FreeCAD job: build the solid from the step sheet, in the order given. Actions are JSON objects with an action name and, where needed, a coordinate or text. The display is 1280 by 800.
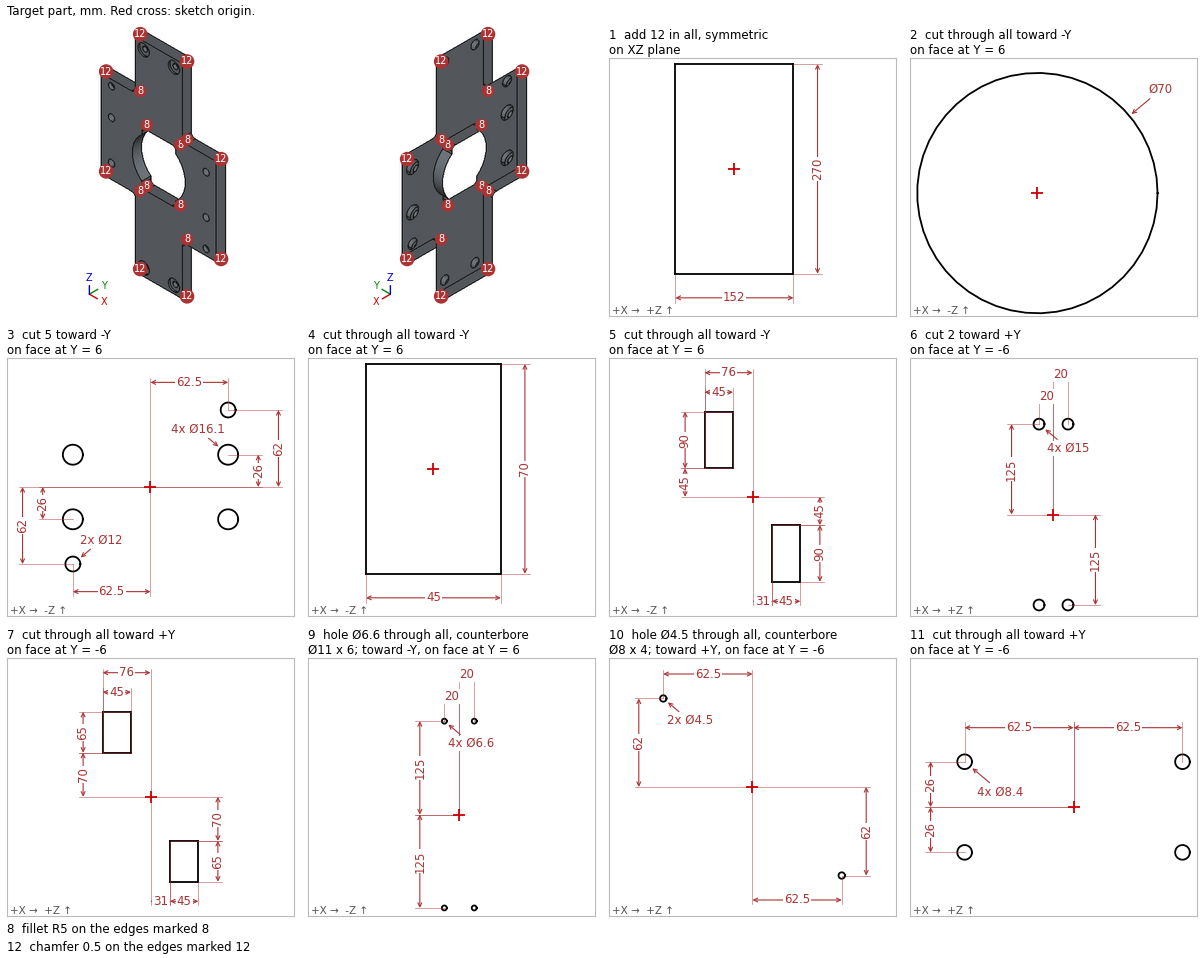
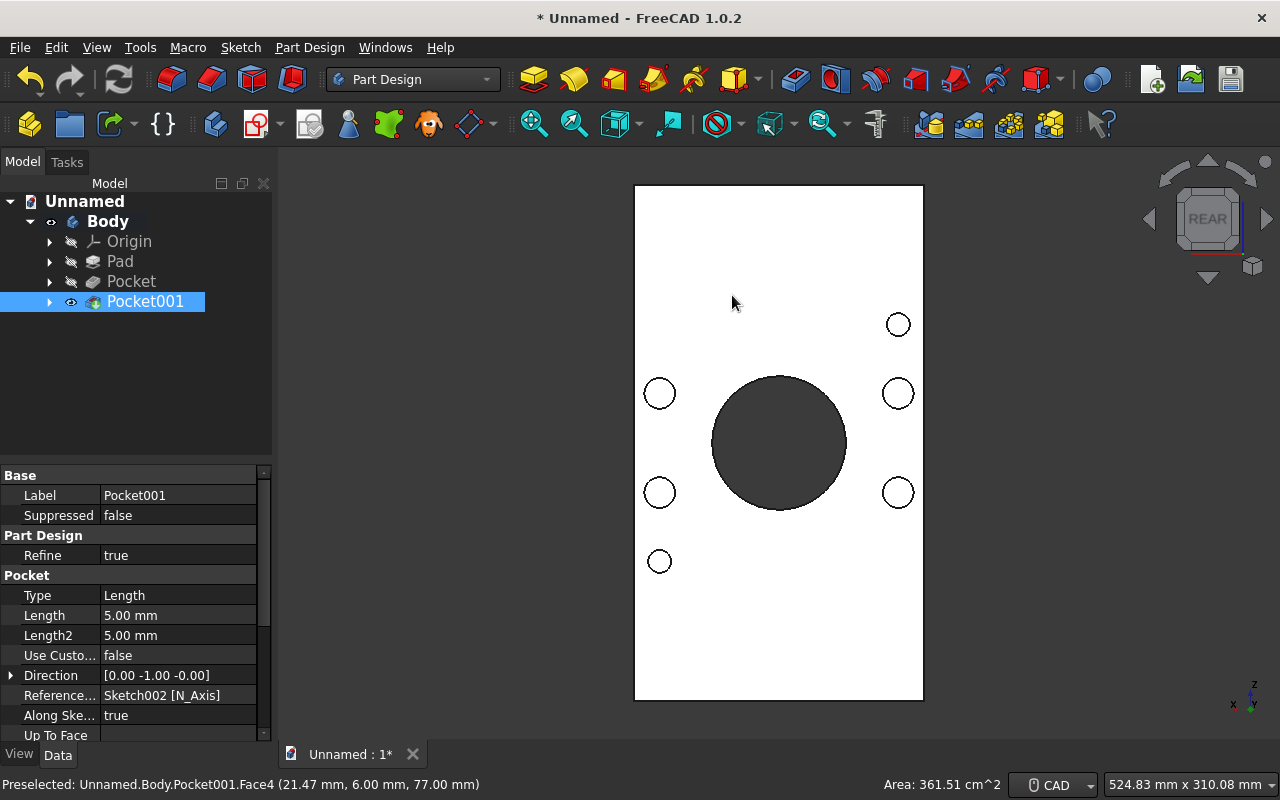
{"action": "left_click", "coordinate": [256, 124]}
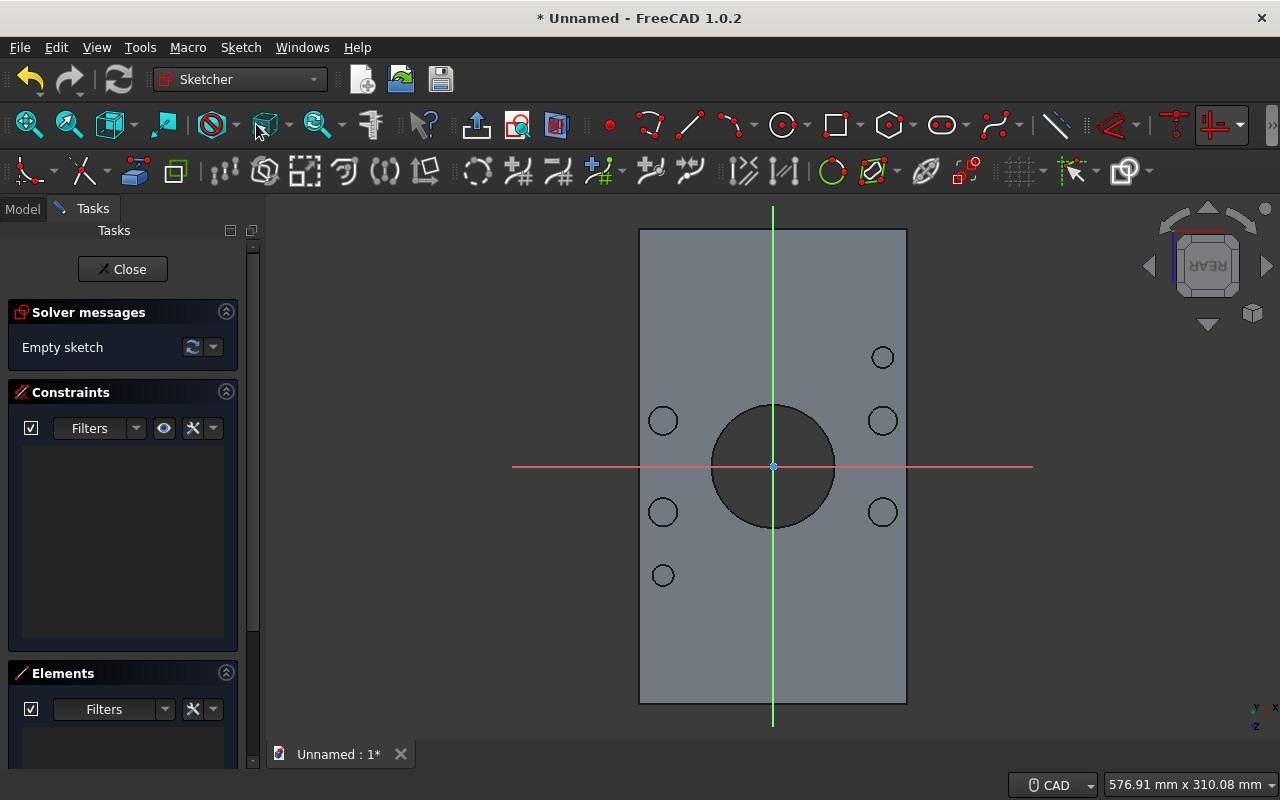
{"action": "scroll", "coordinate": [813, 466], "scroll_direction": "up", "scroll_amount": 5}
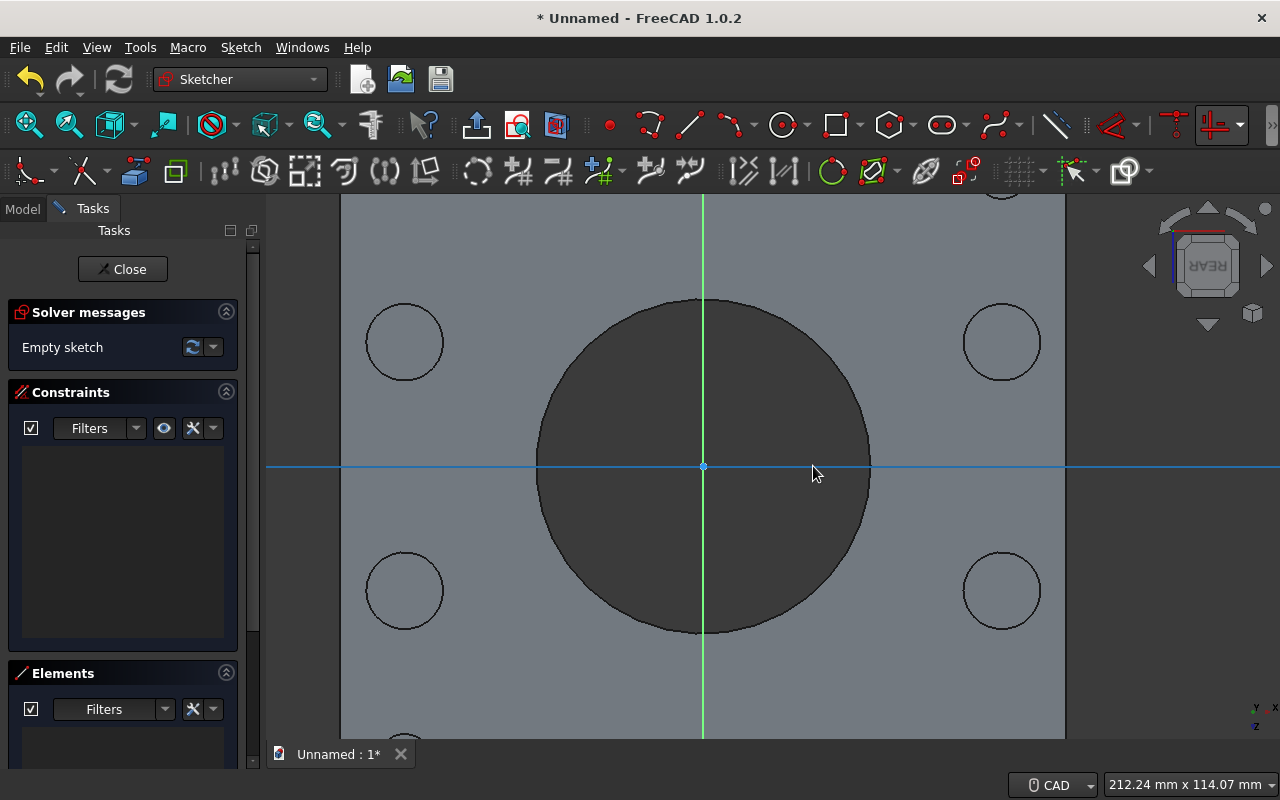
{"action": "left_click", "coordinate": [862, 126]}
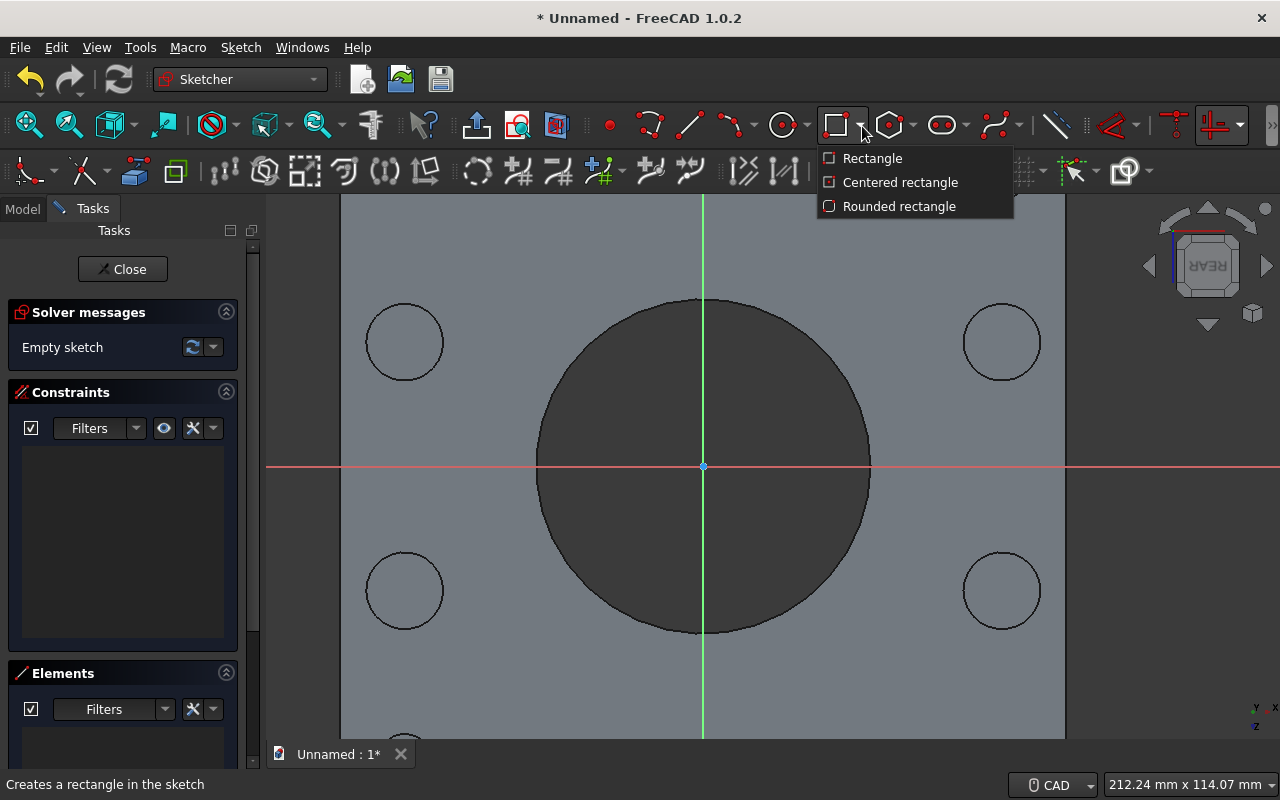
{"action": "left_click", "coordinate": [916, 182]}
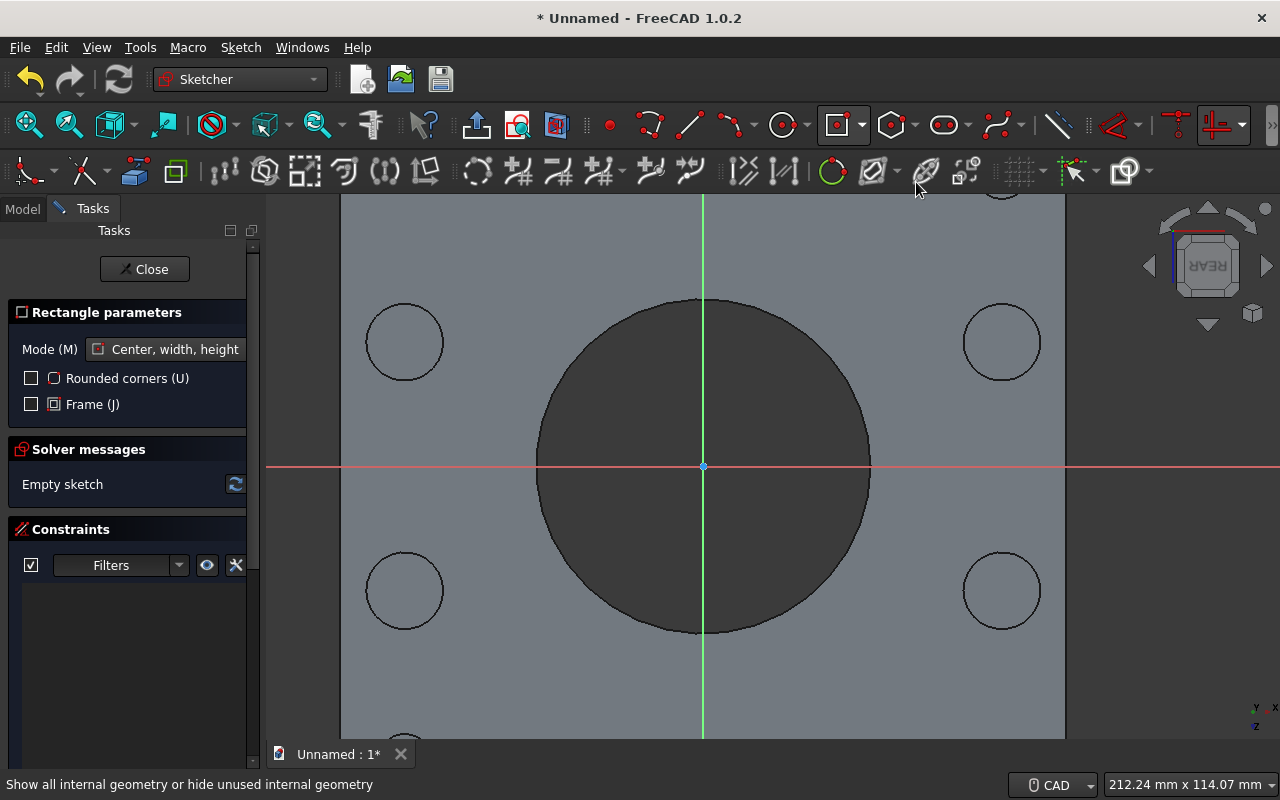
{"action": "left_click", "coordinate": [703, 466]}
{"action": "mouse_move", "coordinate": [811, 299]}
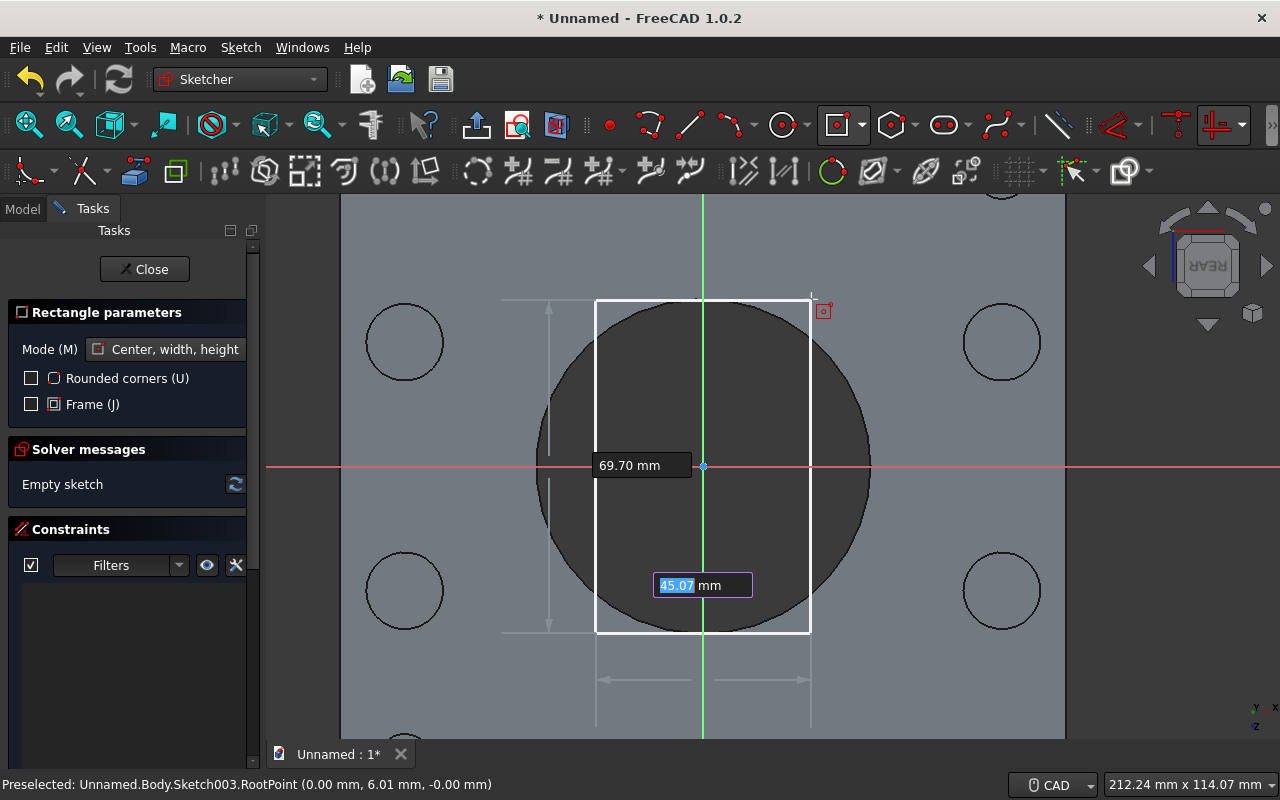
{"action": "type", "text": "45"}
{"action": "key", "text": "Tab"}
{"action": "type", "text": "70"}
{"action": "key", "text": "Return"}
{"action": "key", "text": "Escape"}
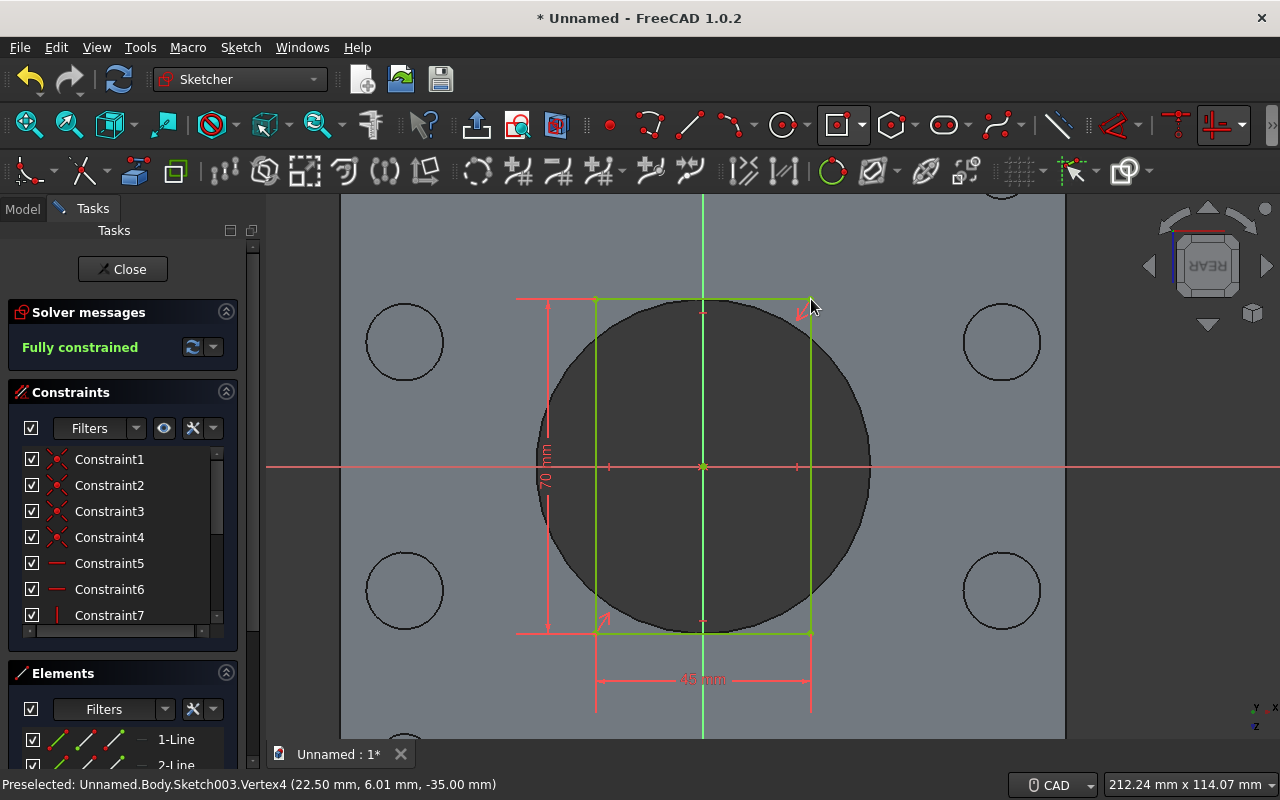
{"action": "left_click", "coordinate": [123, 269]}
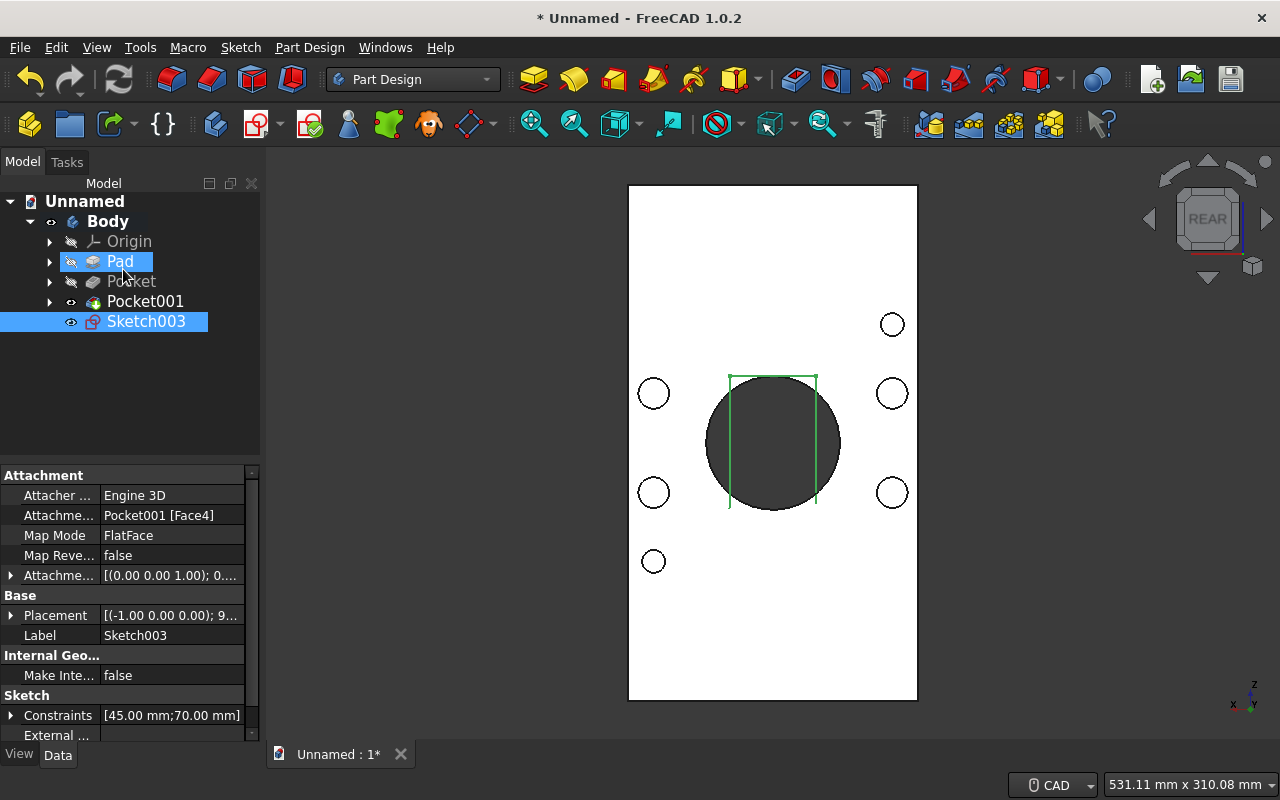
{"action": "left_click", "coordinate": [796, 80]}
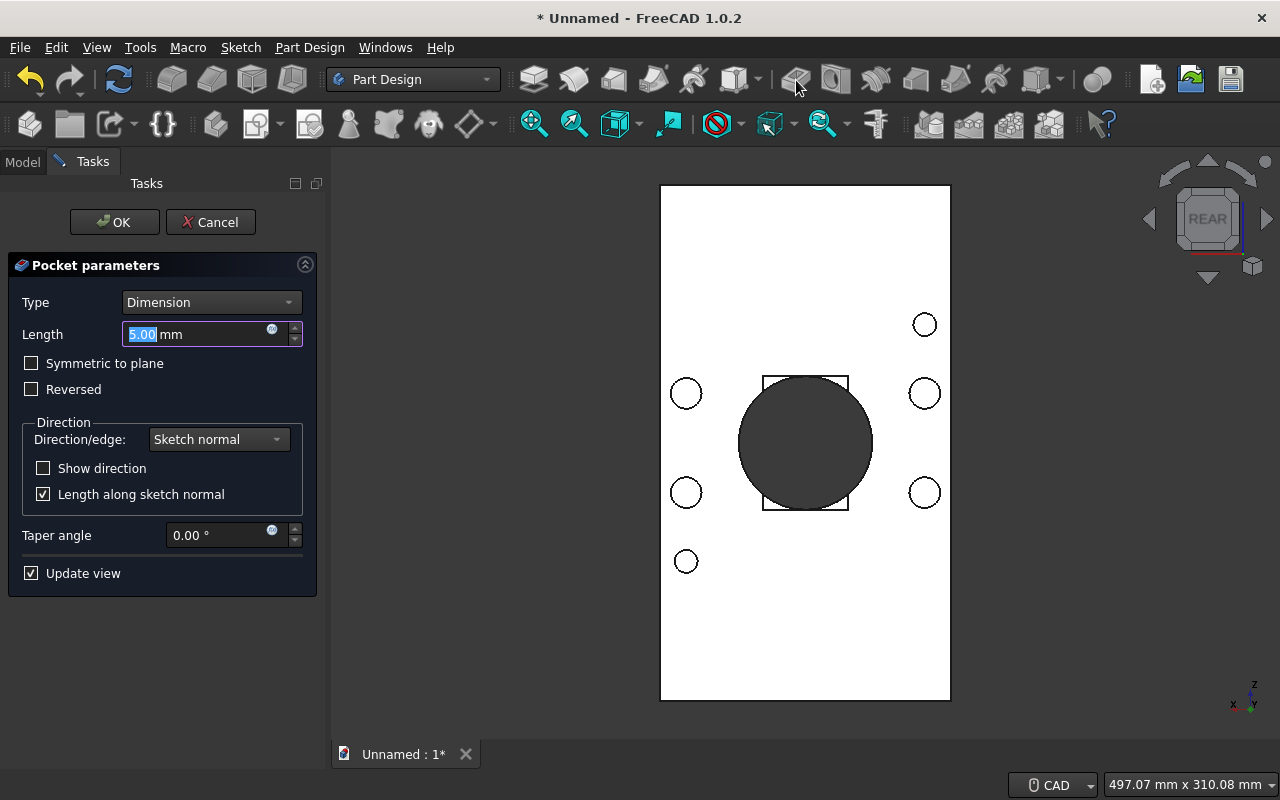
{"action": "left_click", "coordinate": [212, 302]}